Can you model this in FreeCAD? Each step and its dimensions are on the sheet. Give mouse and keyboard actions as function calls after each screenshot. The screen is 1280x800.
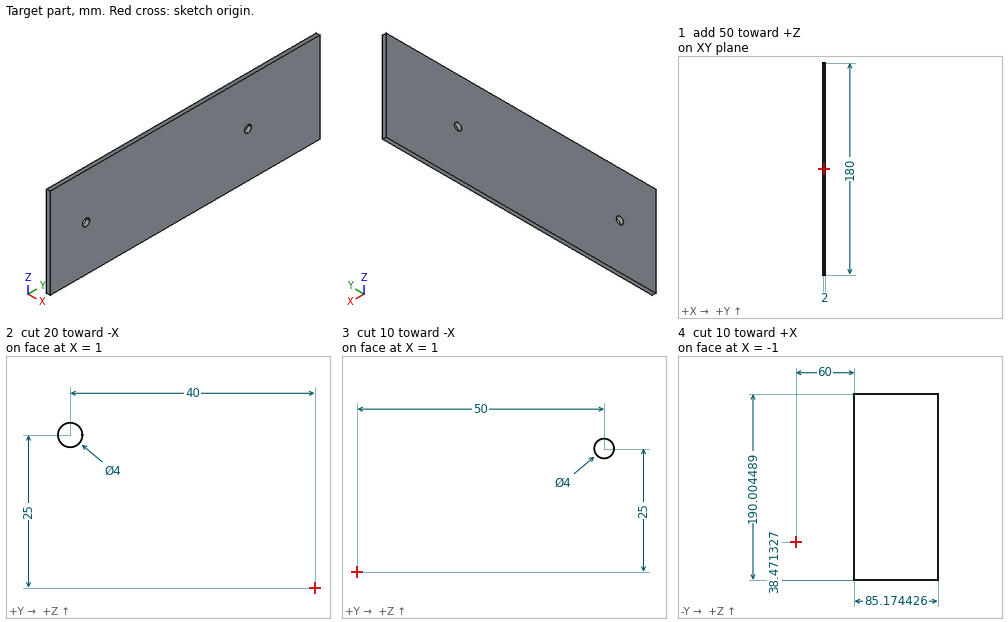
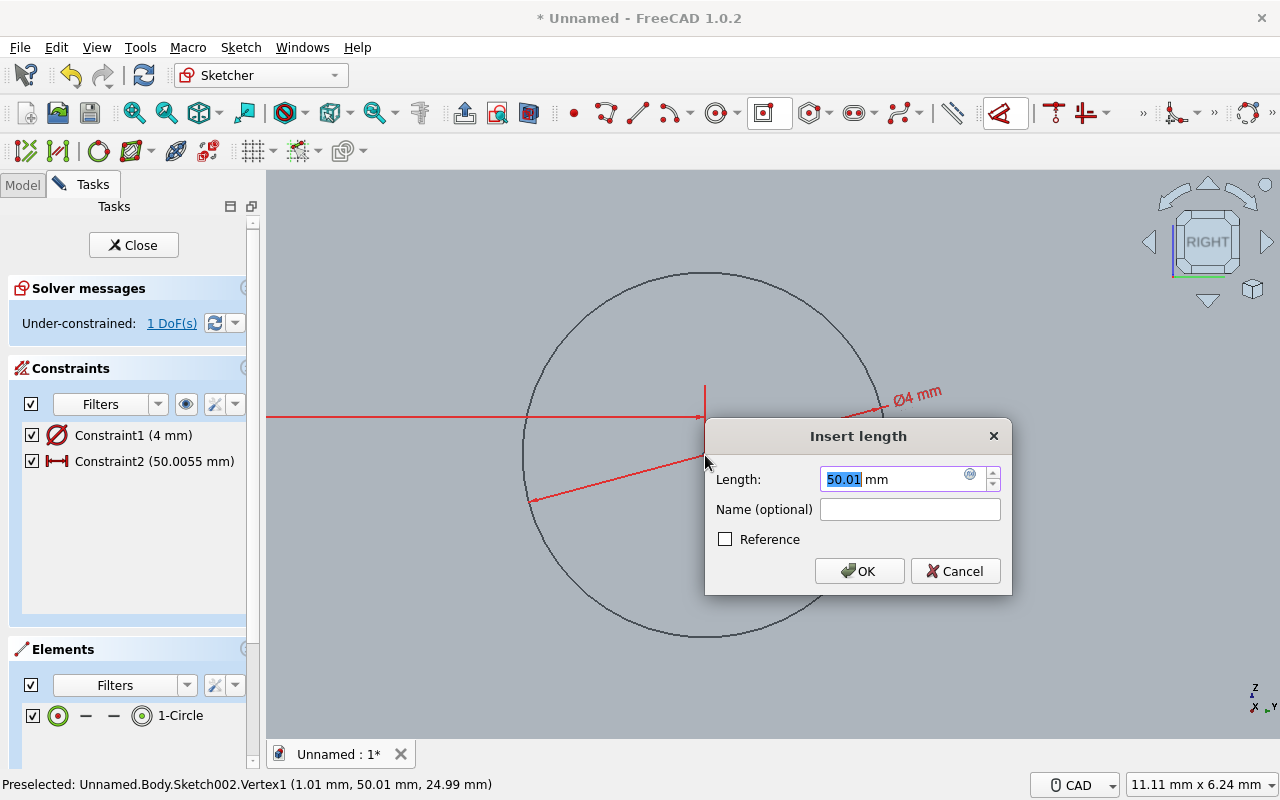
text(50)
key(Return)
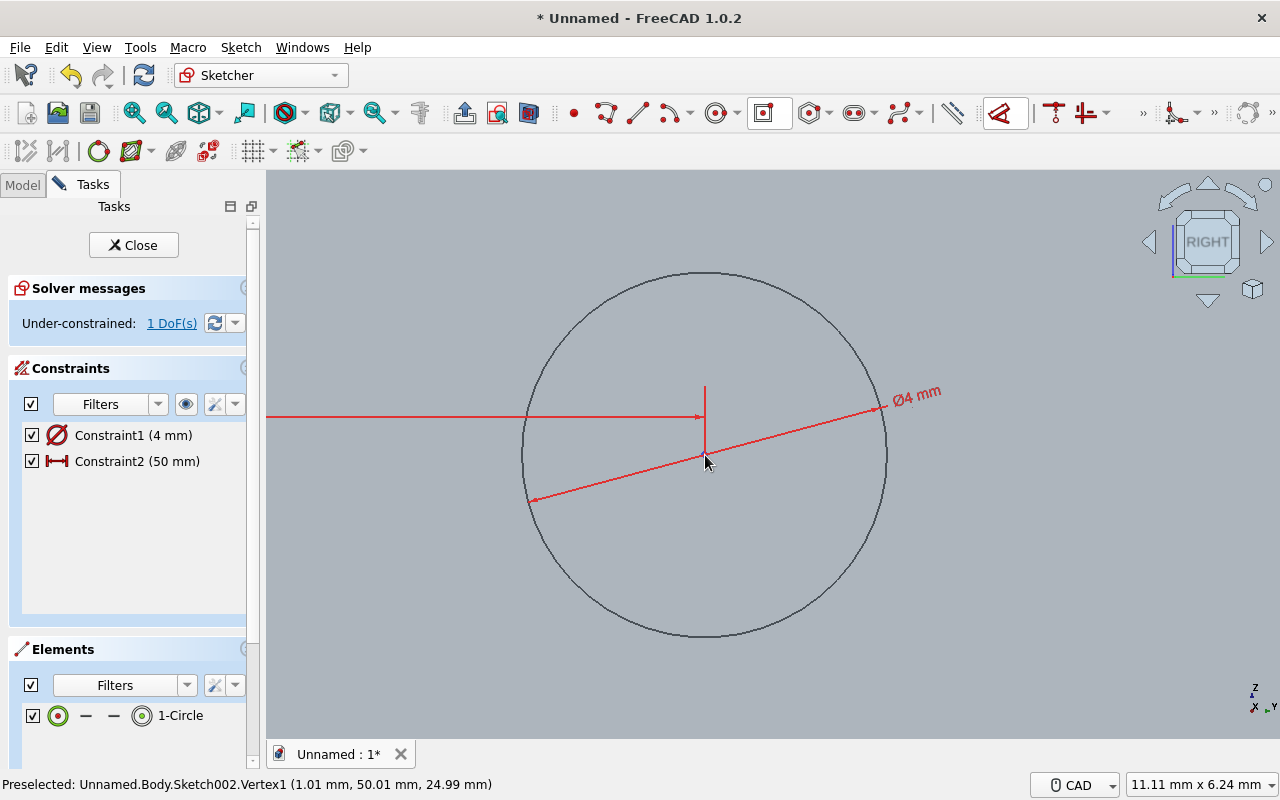
click(705, 455)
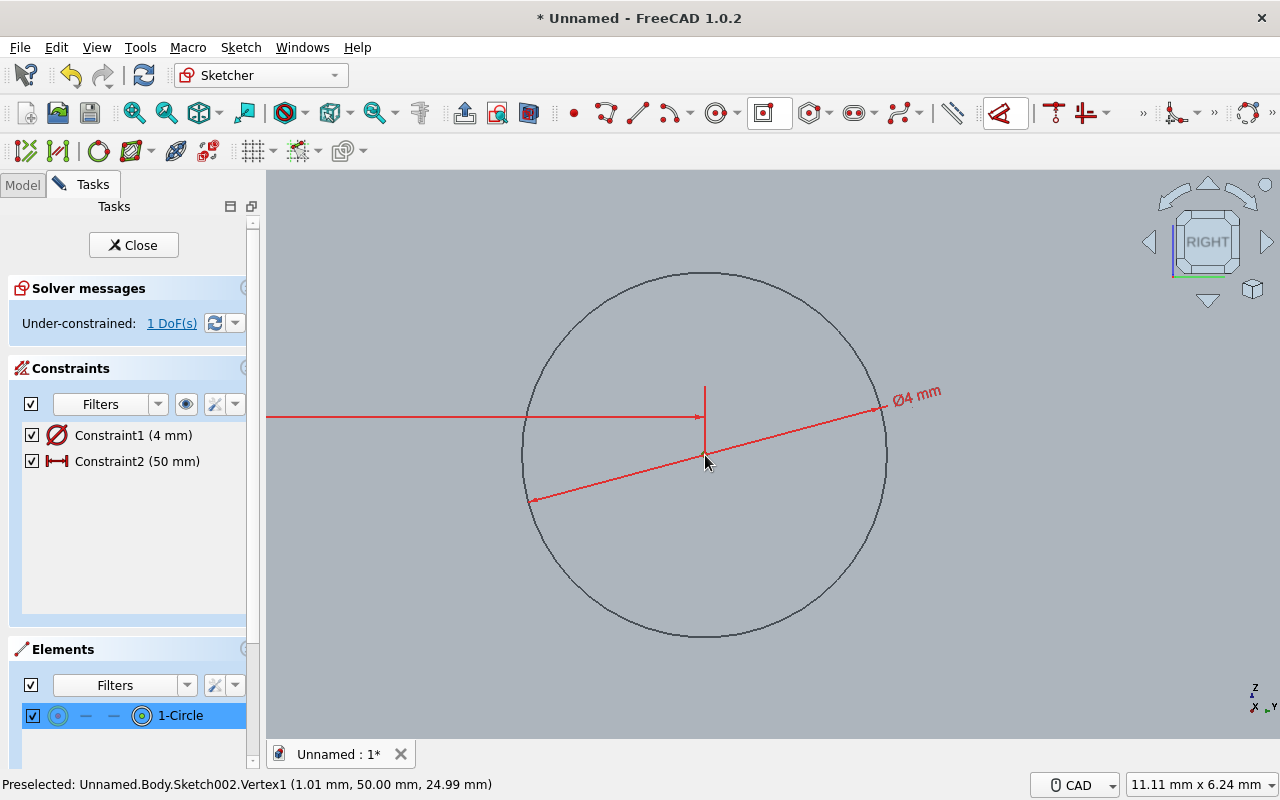
click(1022, 114)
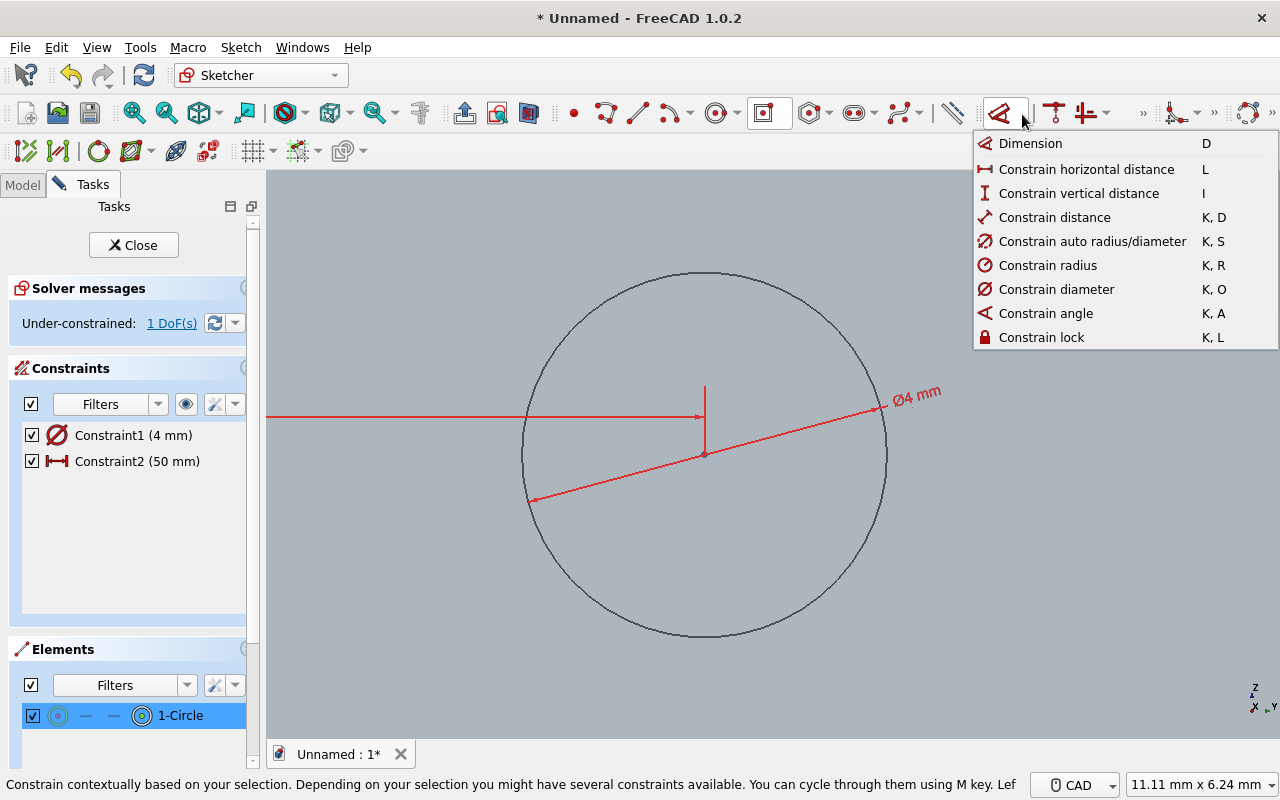
click(1126, 193)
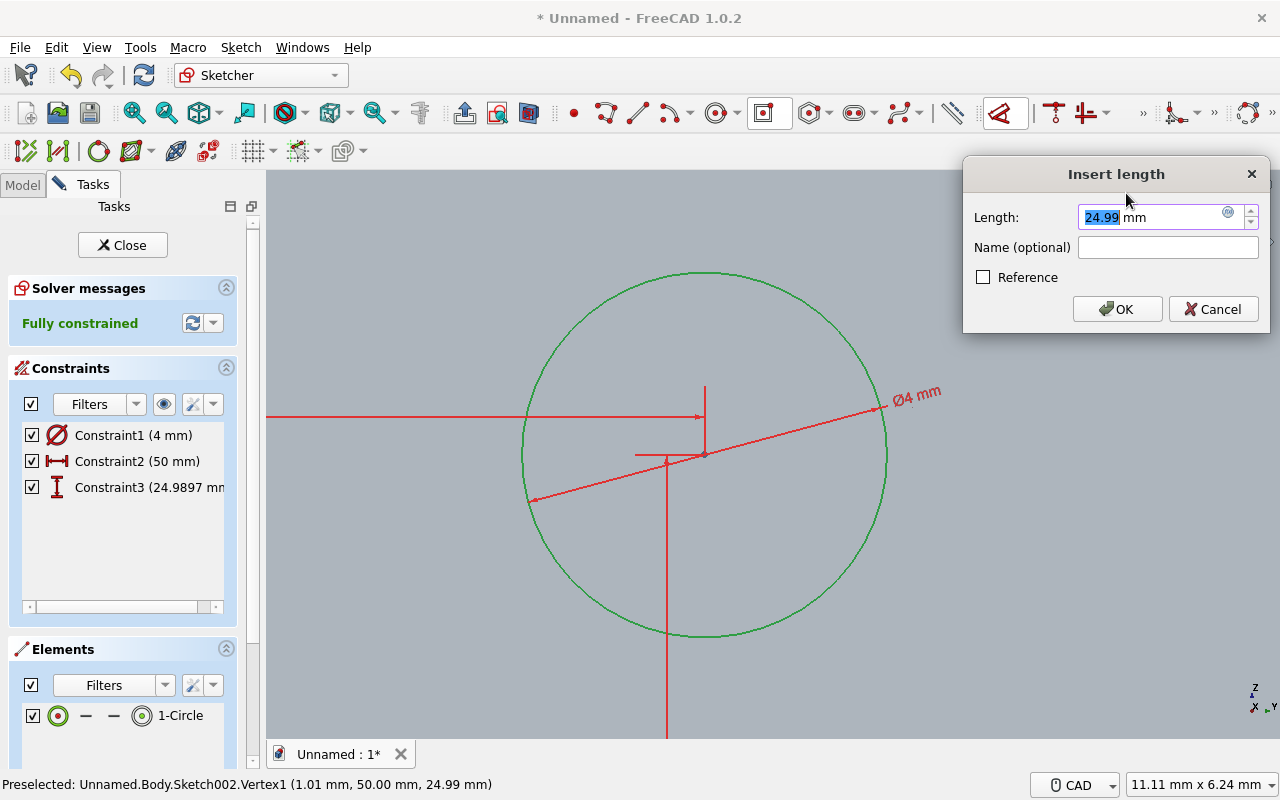
text(25)
key(Return)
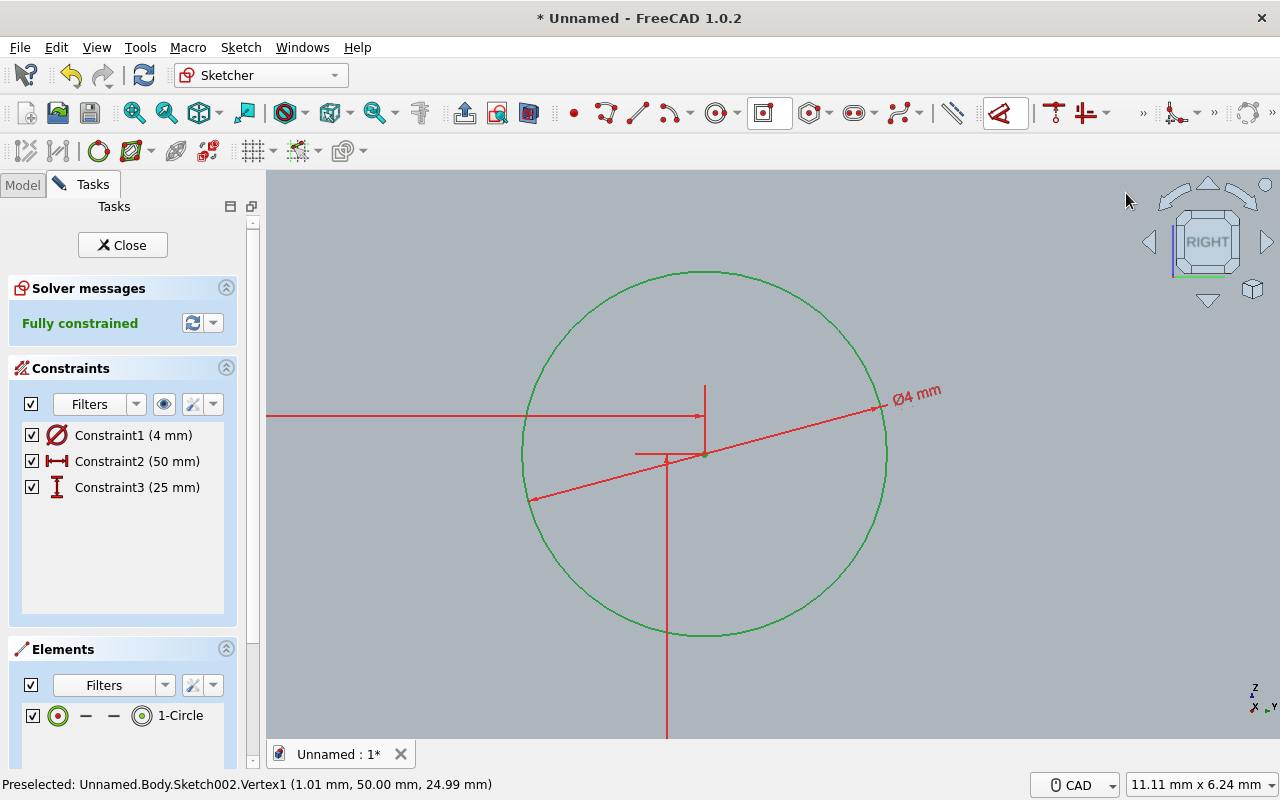
click(123, 245)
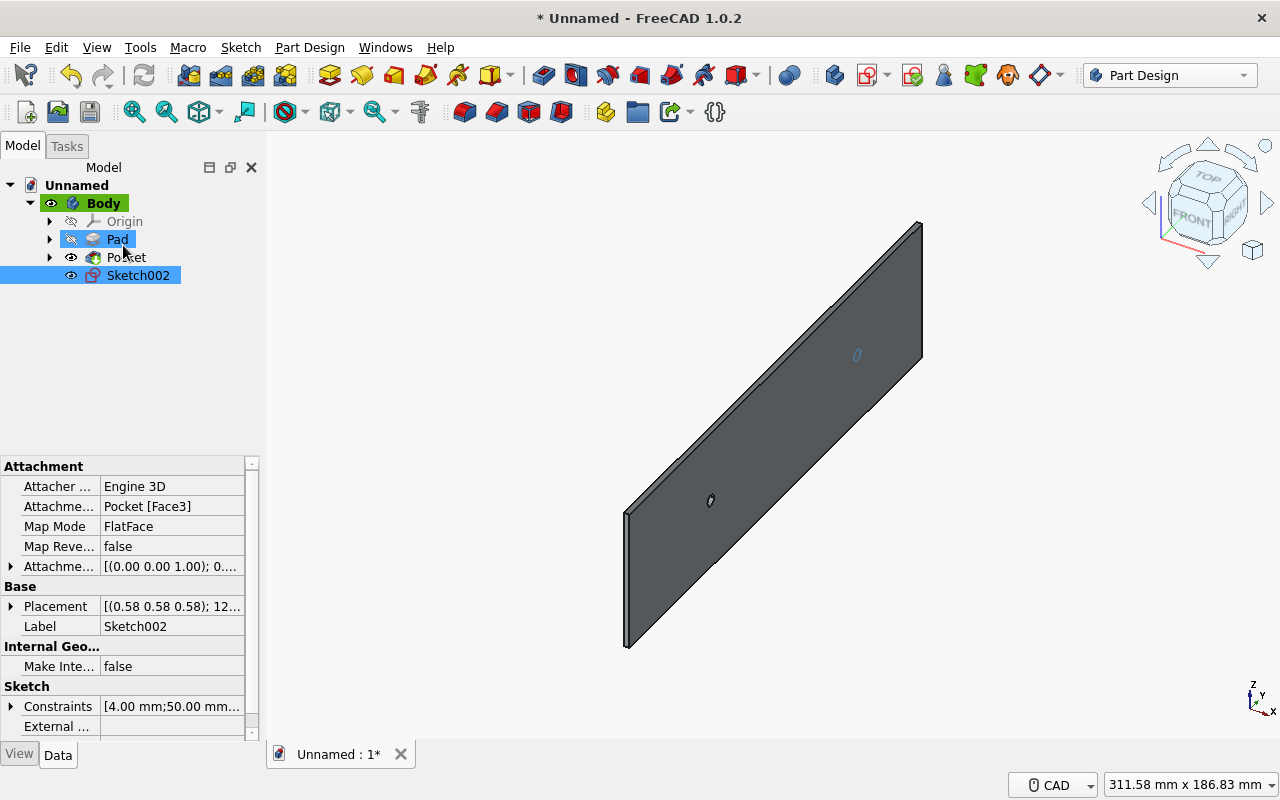
click(544, 76)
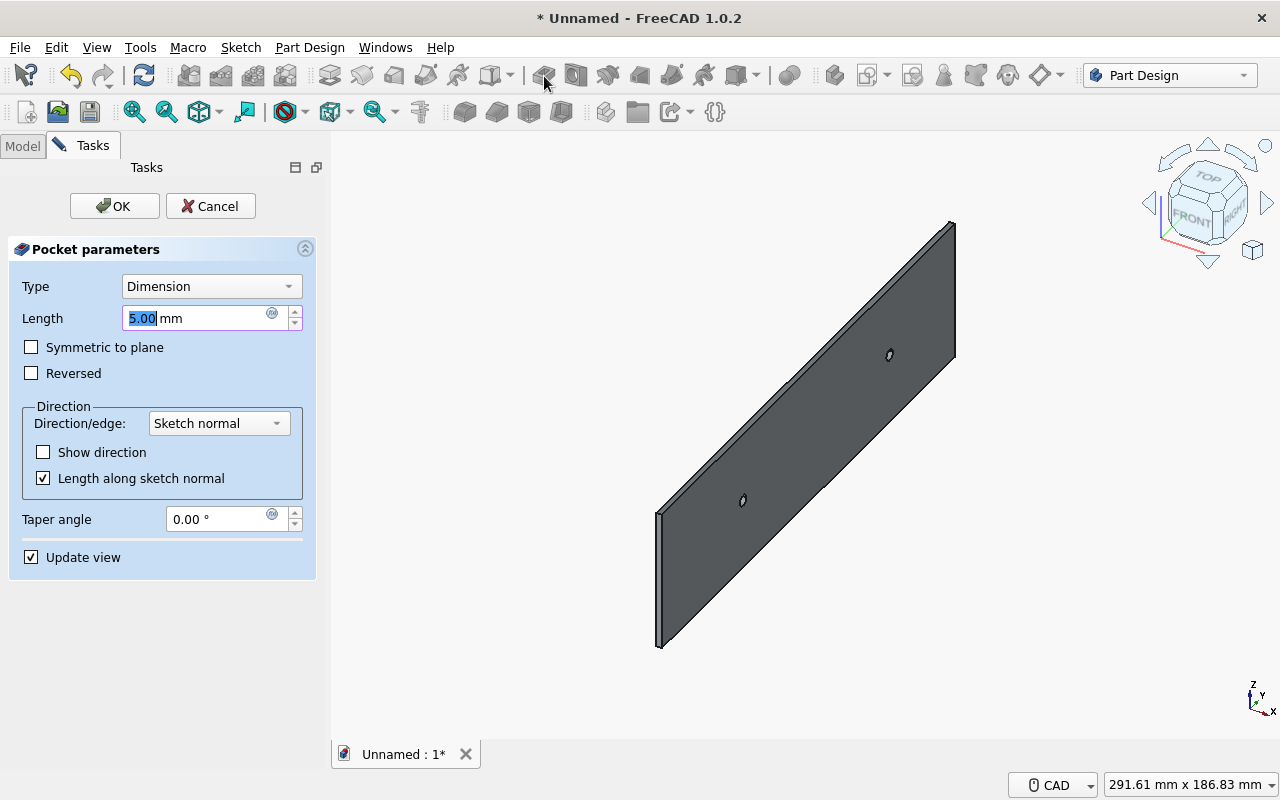
text(10)
key(Tab)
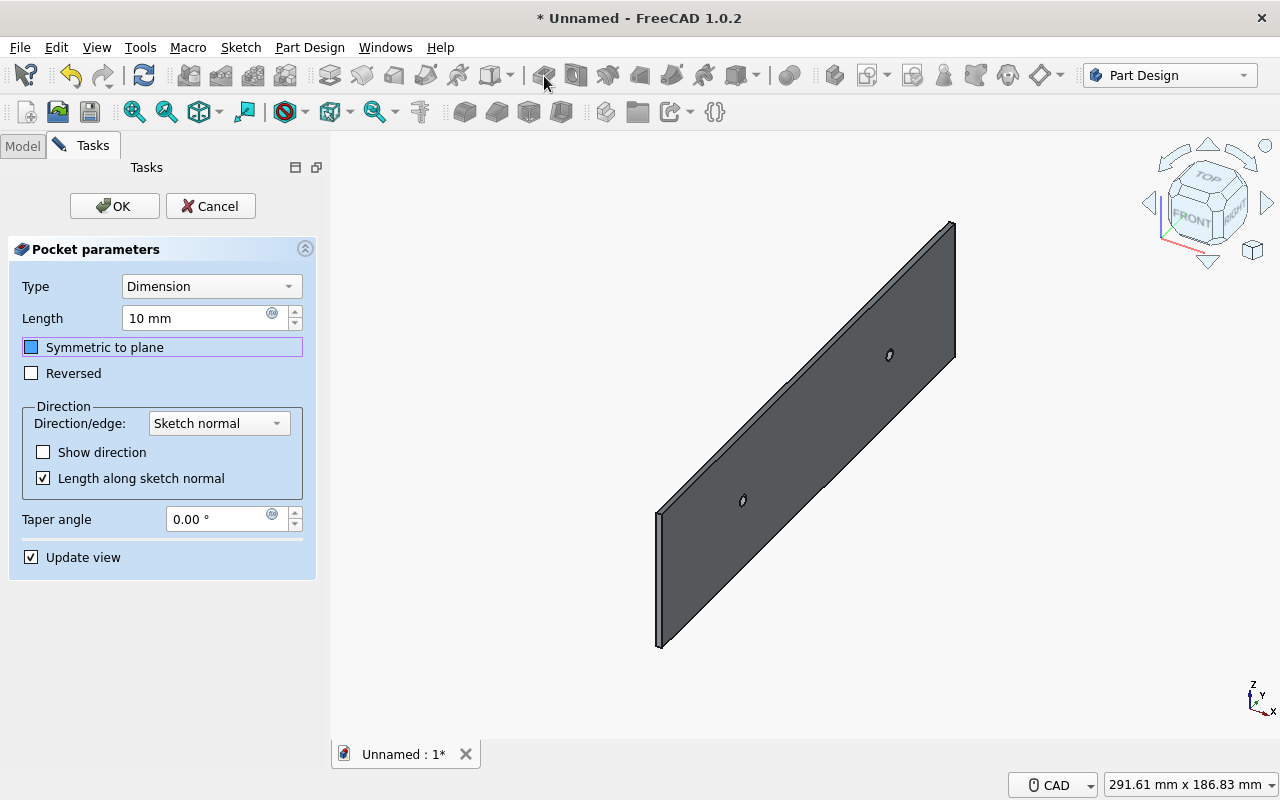
click(115, 206)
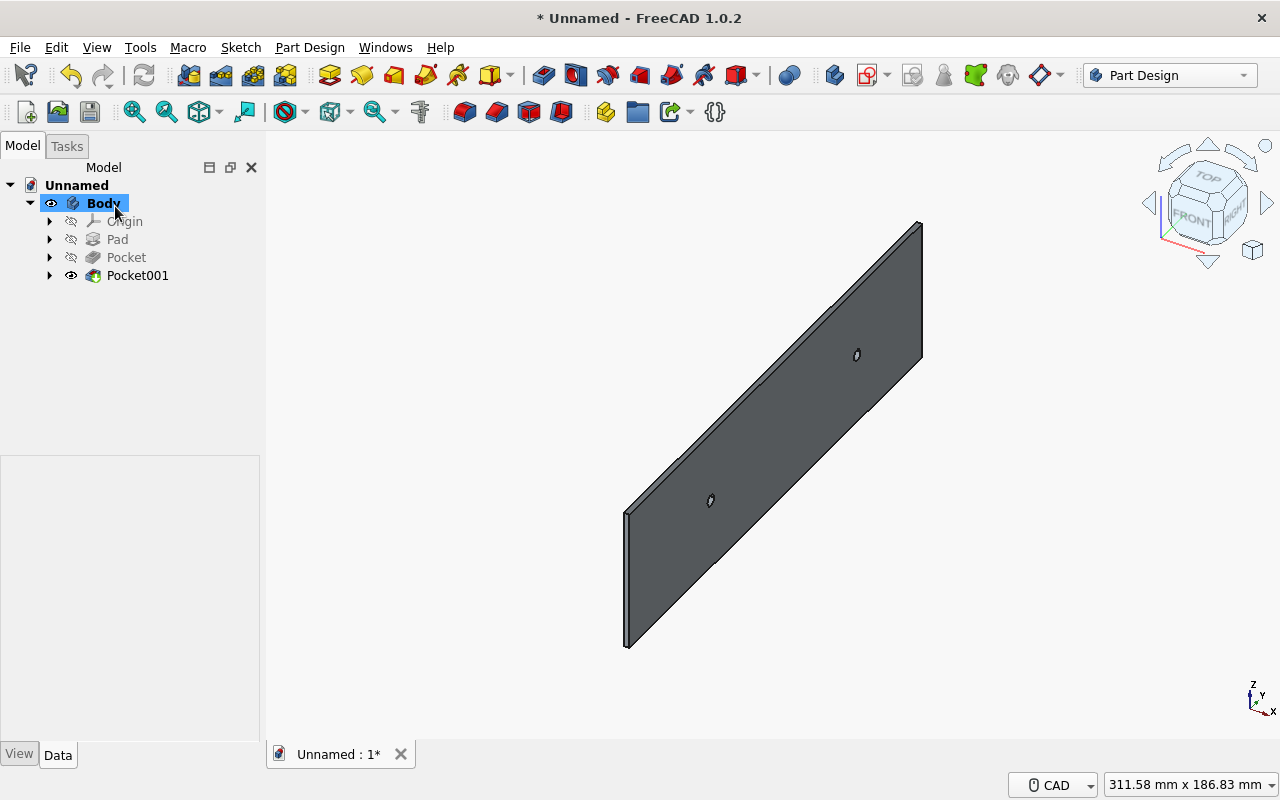
key(6)